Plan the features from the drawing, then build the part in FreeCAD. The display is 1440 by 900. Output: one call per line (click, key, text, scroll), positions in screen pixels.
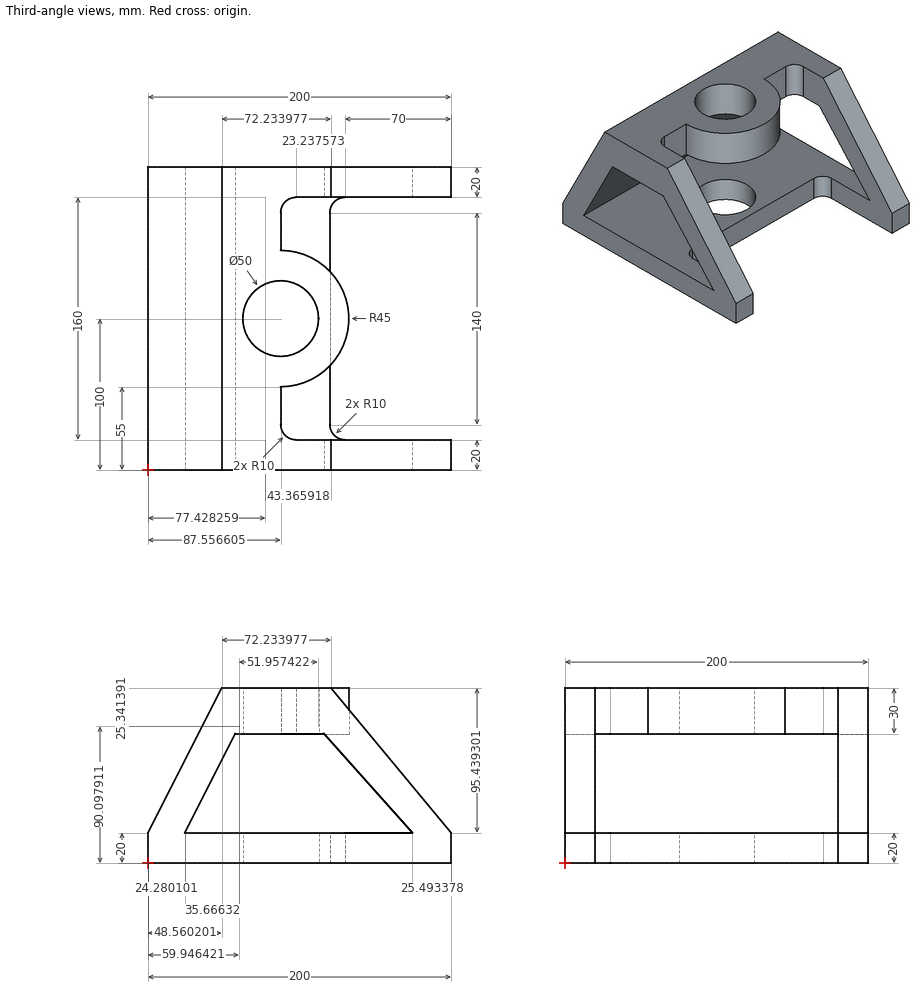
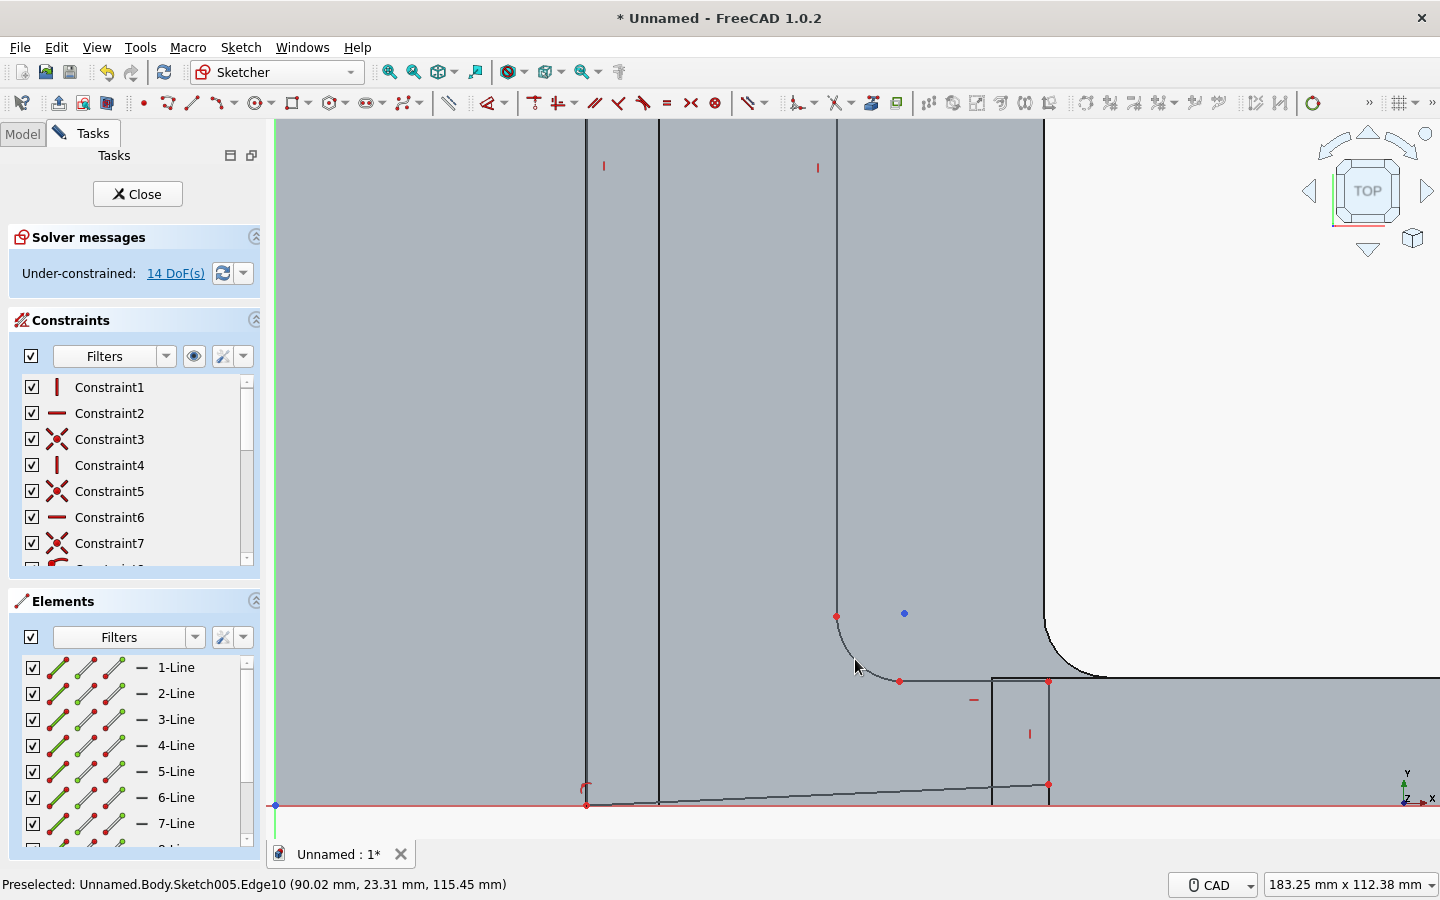
click(837, 347)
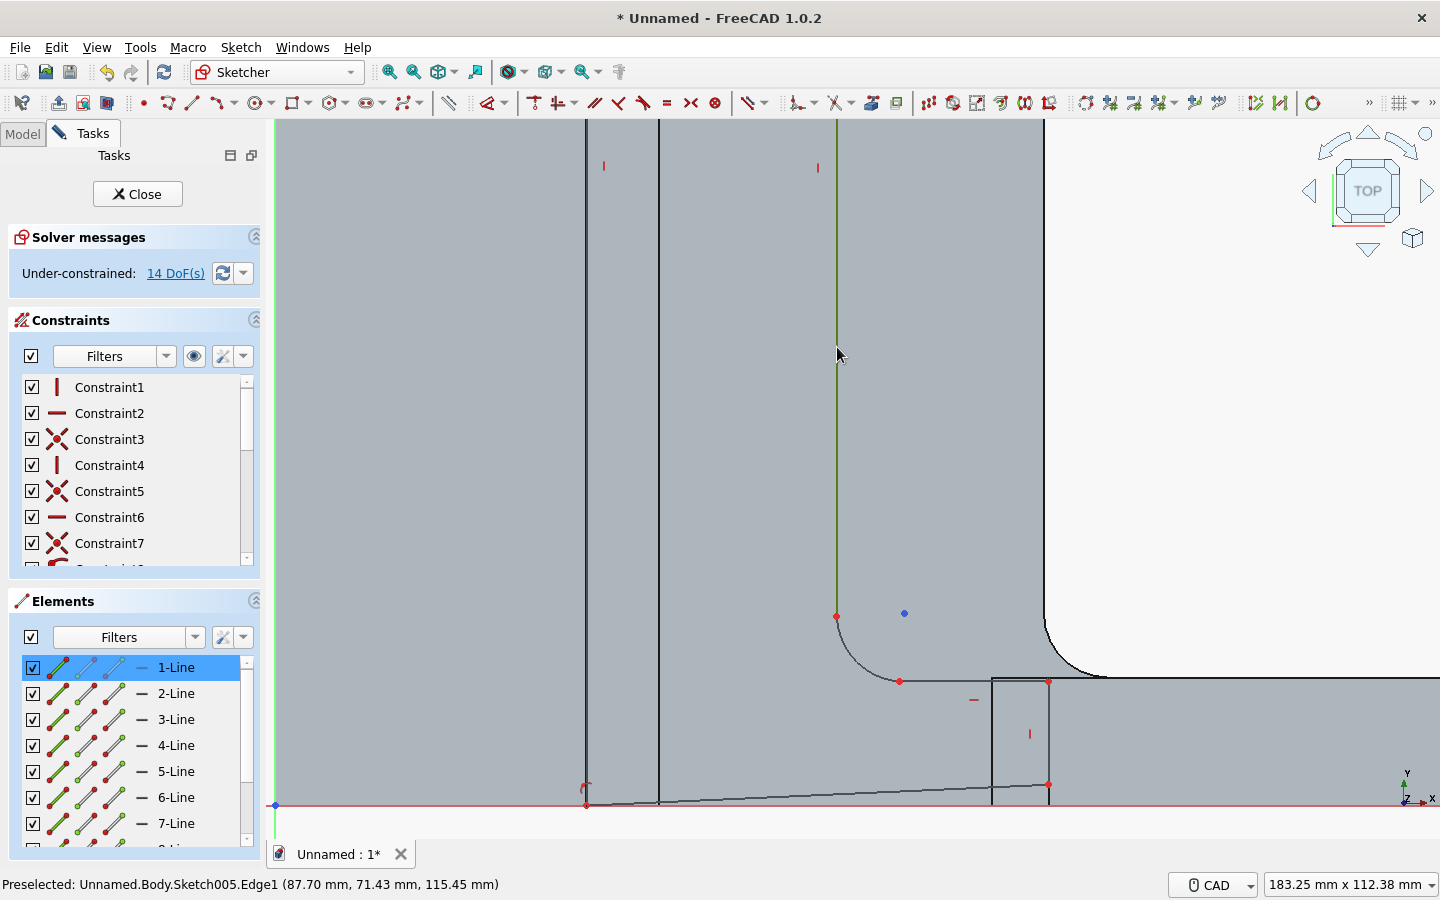
scroll(856, 662, down, 5)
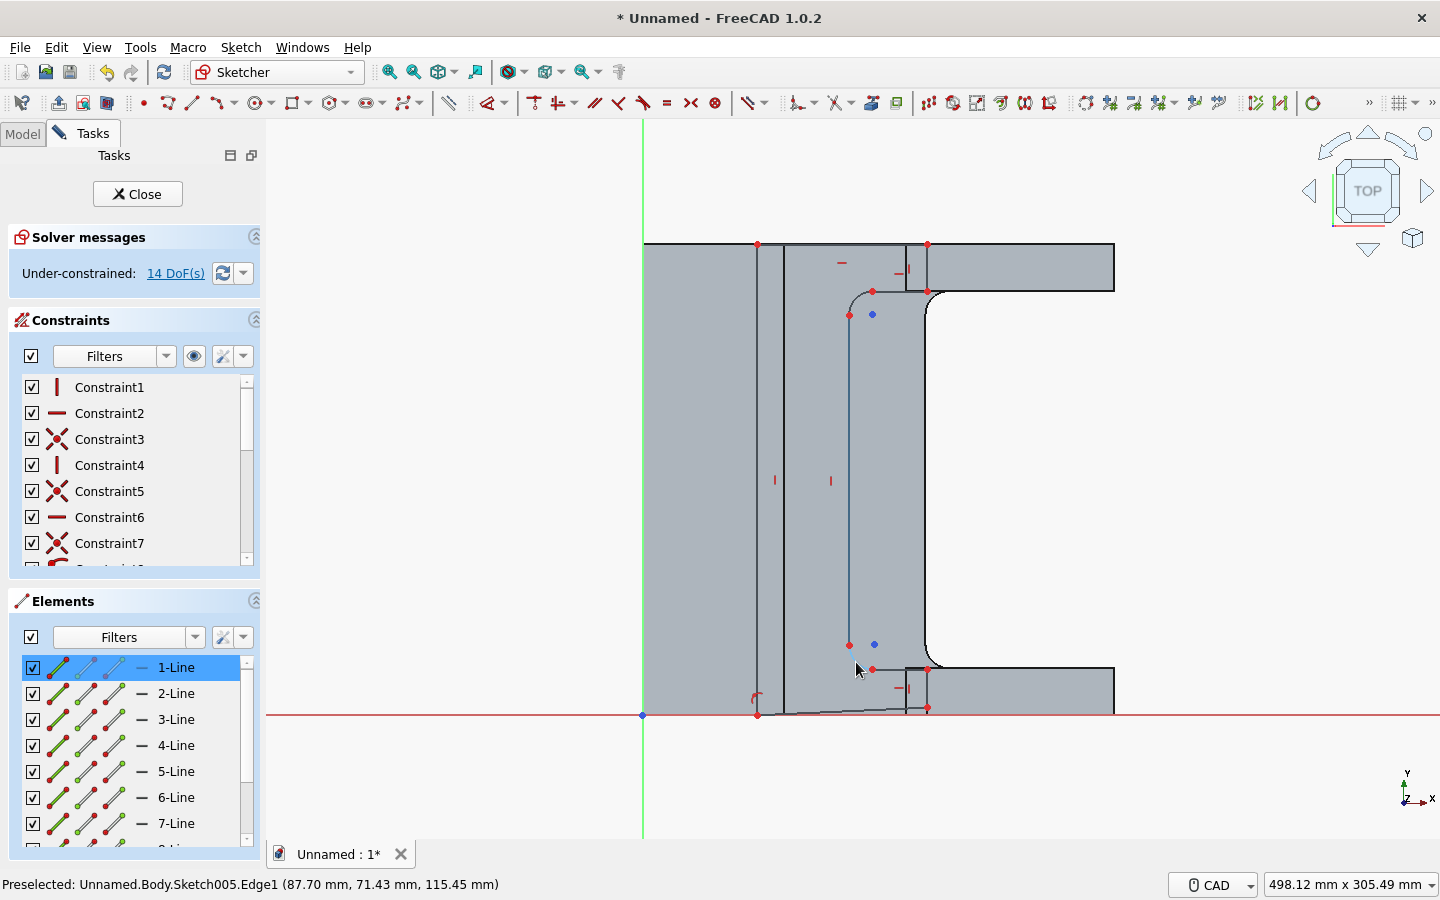
scroll(862, 294, up, 2)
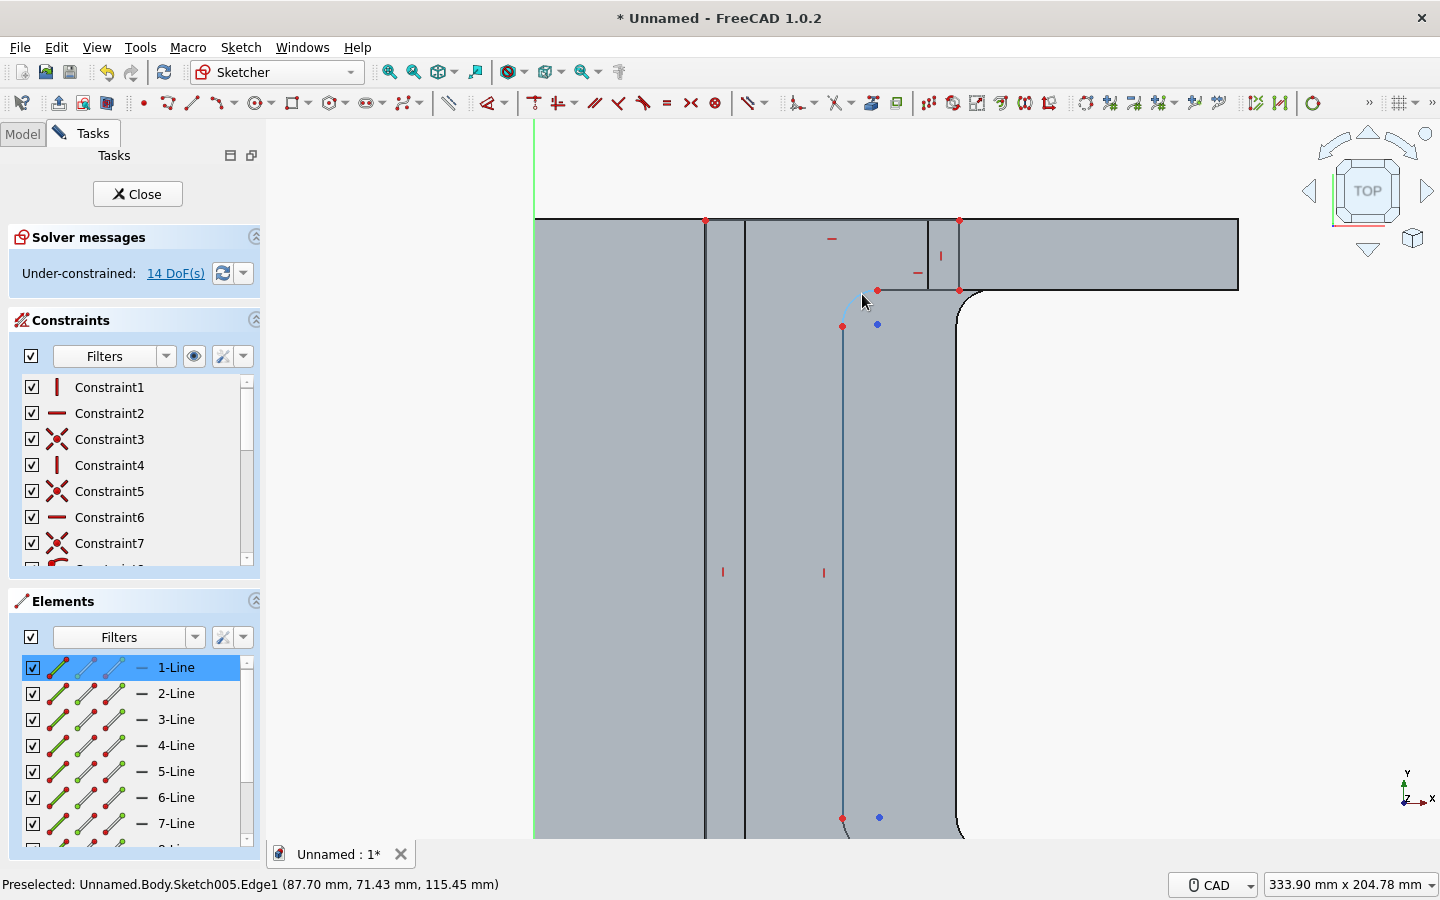
click(861, 294)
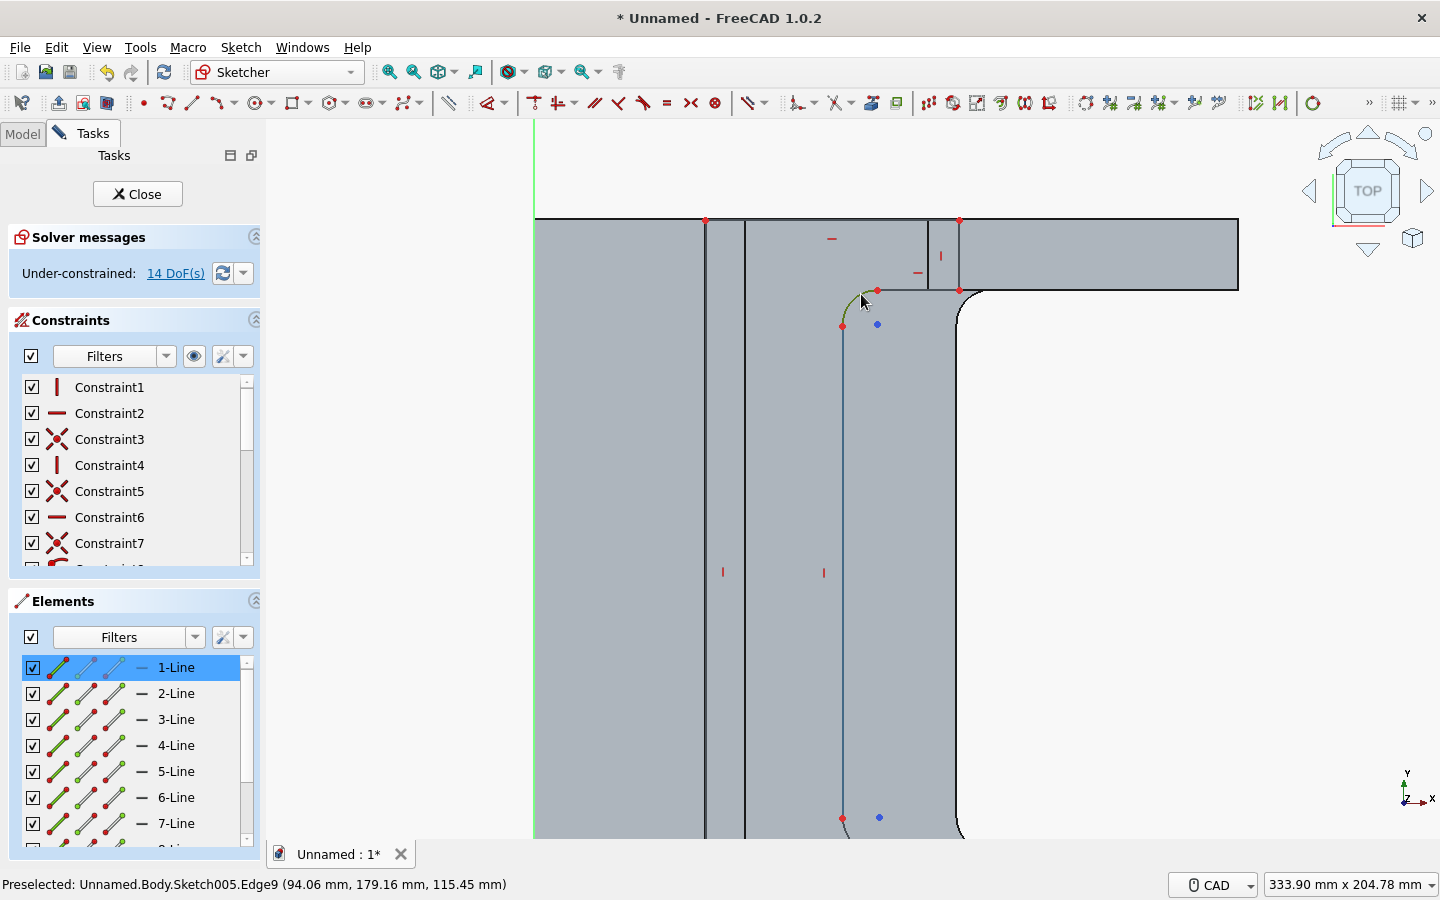
key(t)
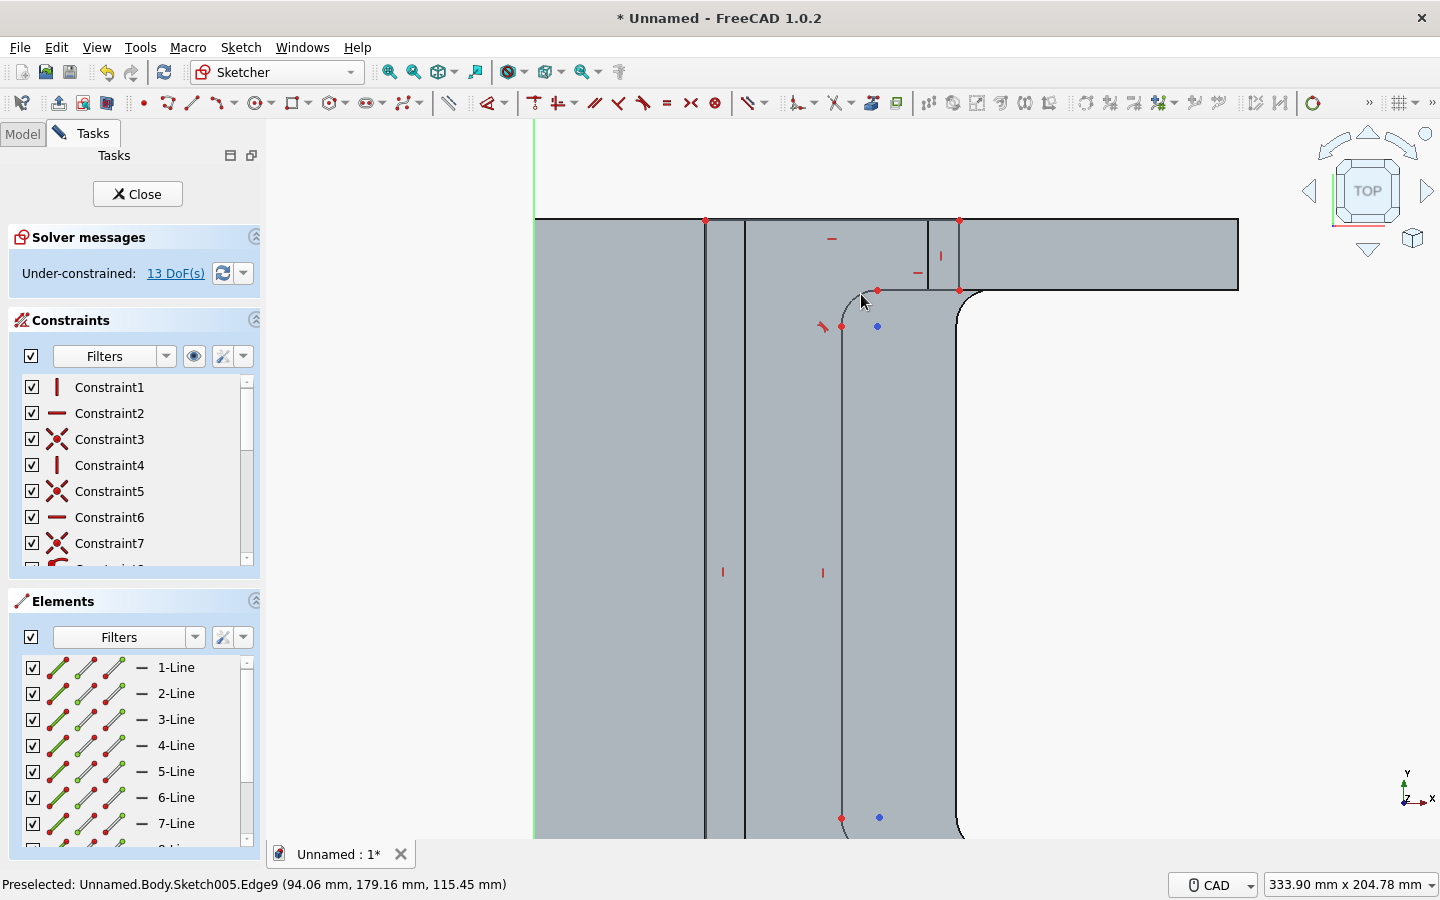
click(842, 671)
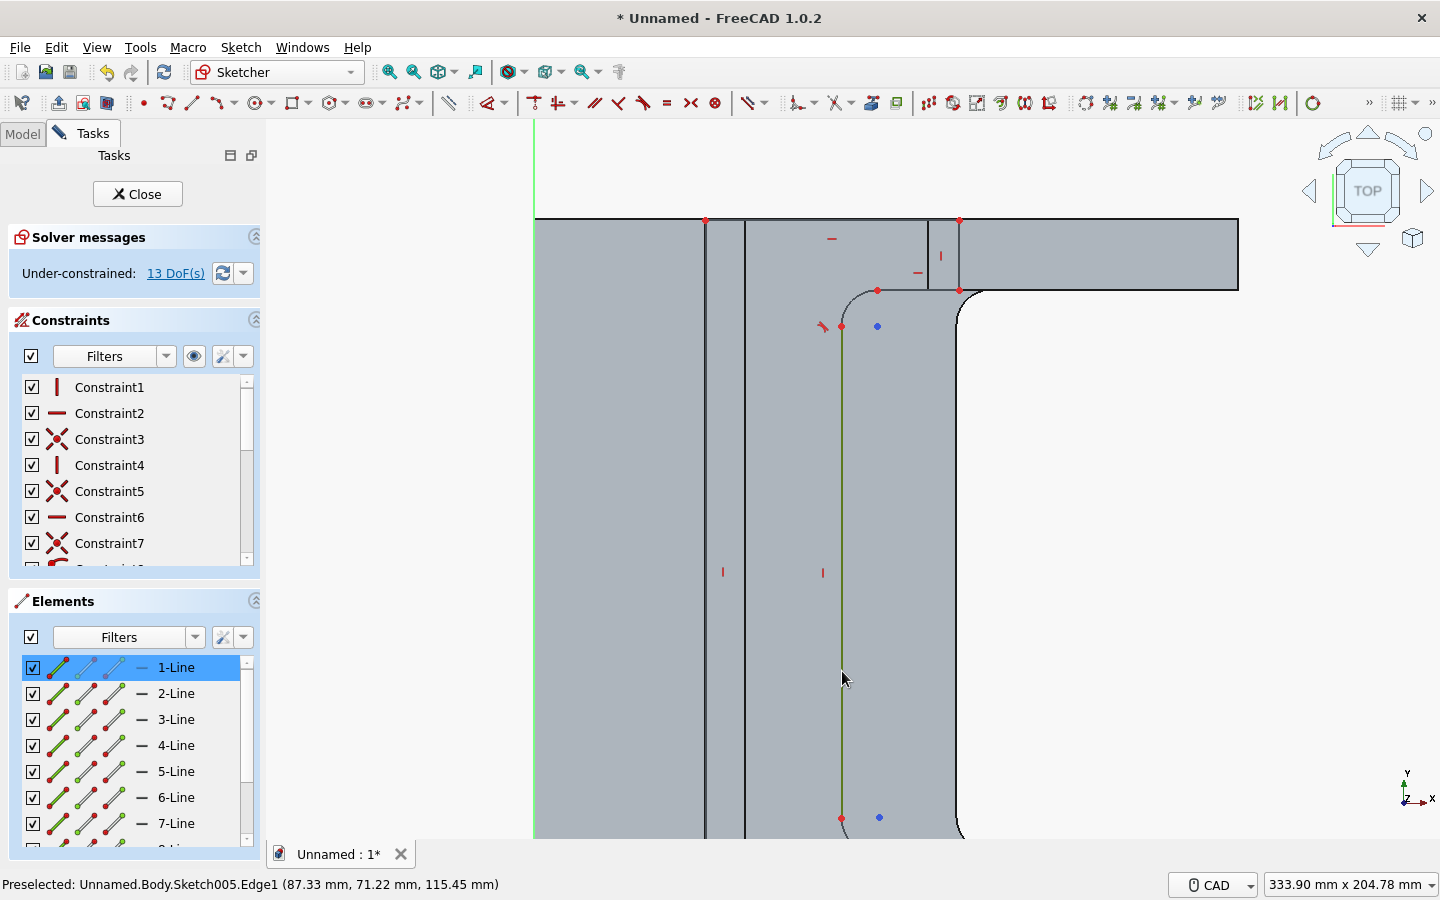
scroll(861, 292, down, 2)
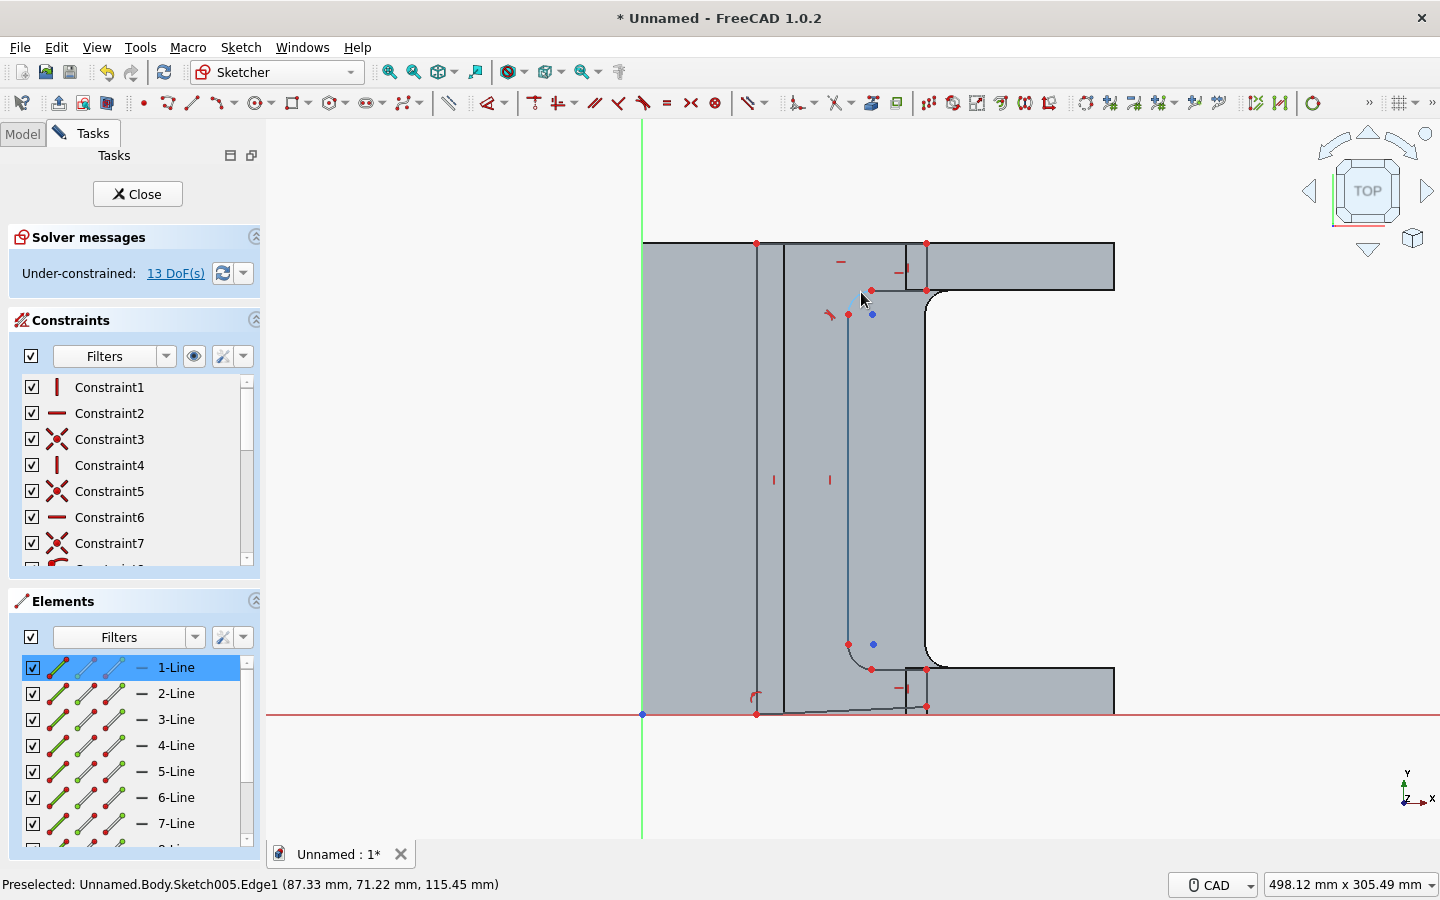
scroll(851, 656, up, 2)